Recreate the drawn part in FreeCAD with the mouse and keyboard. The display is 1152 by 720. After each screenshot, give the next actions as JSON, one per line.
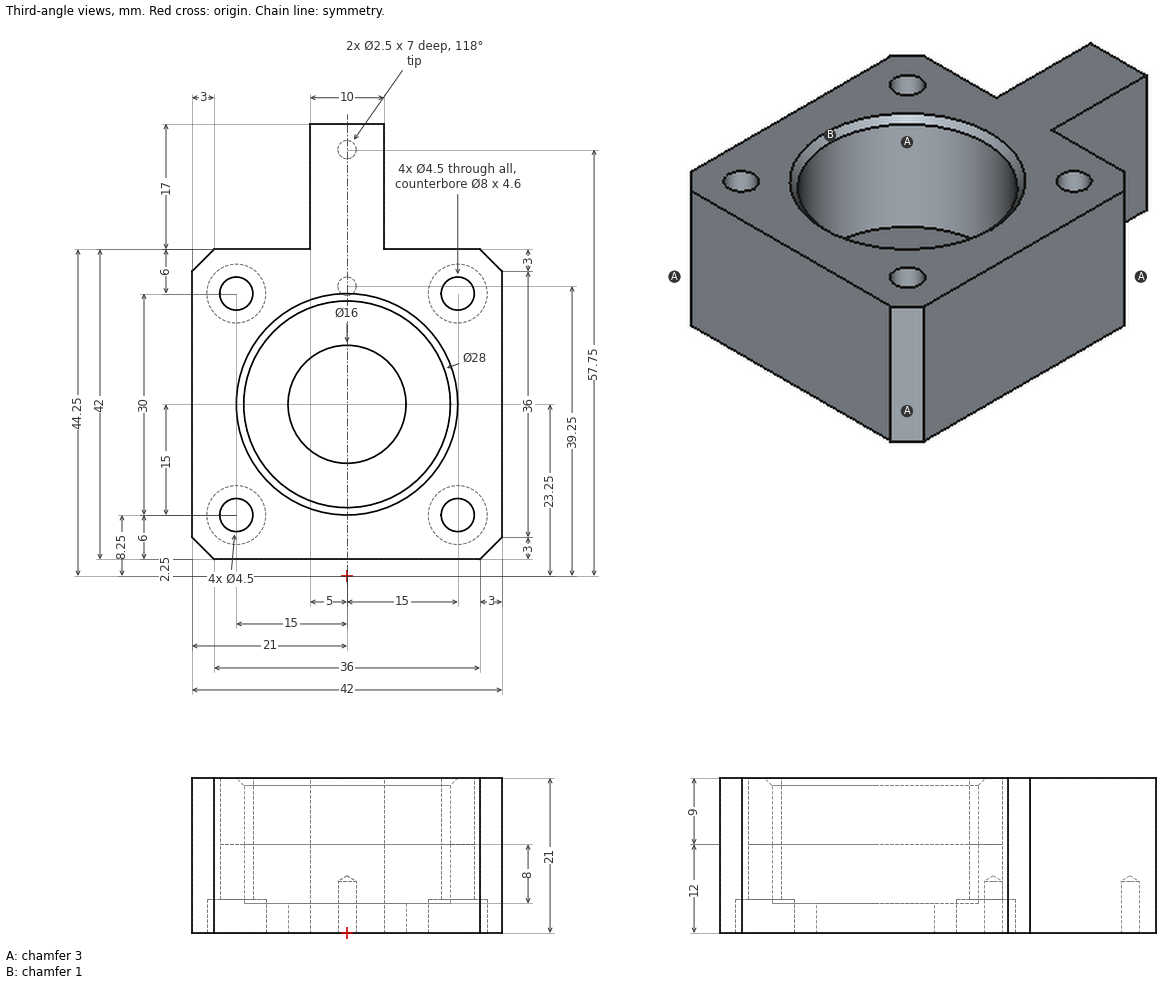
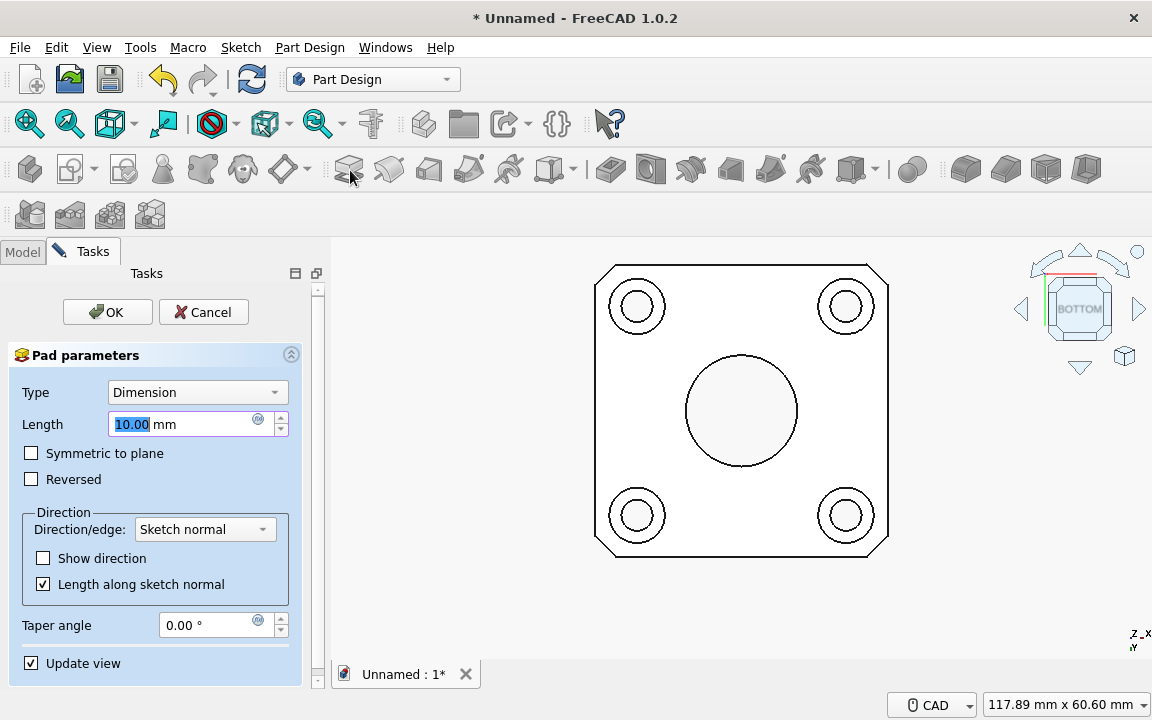
{"action": "type", "text": "21"}
{"action": "key", "text": "Tab"}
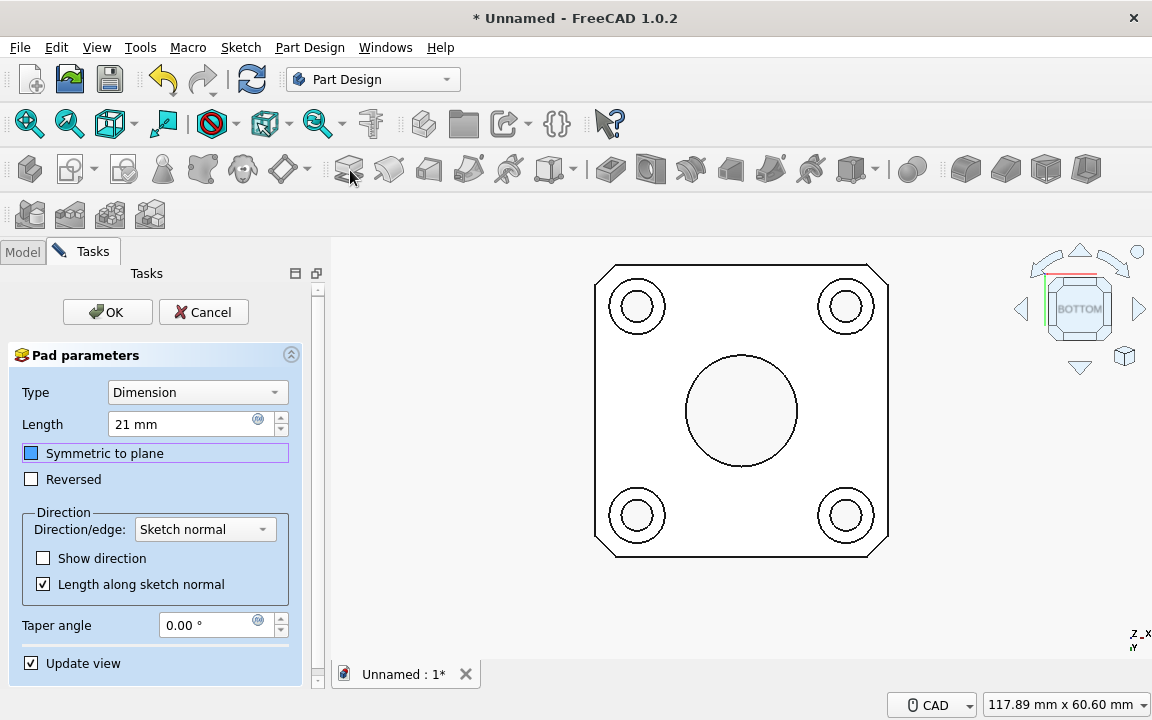
{"action": "left_click", "coordinate": [30, 479]}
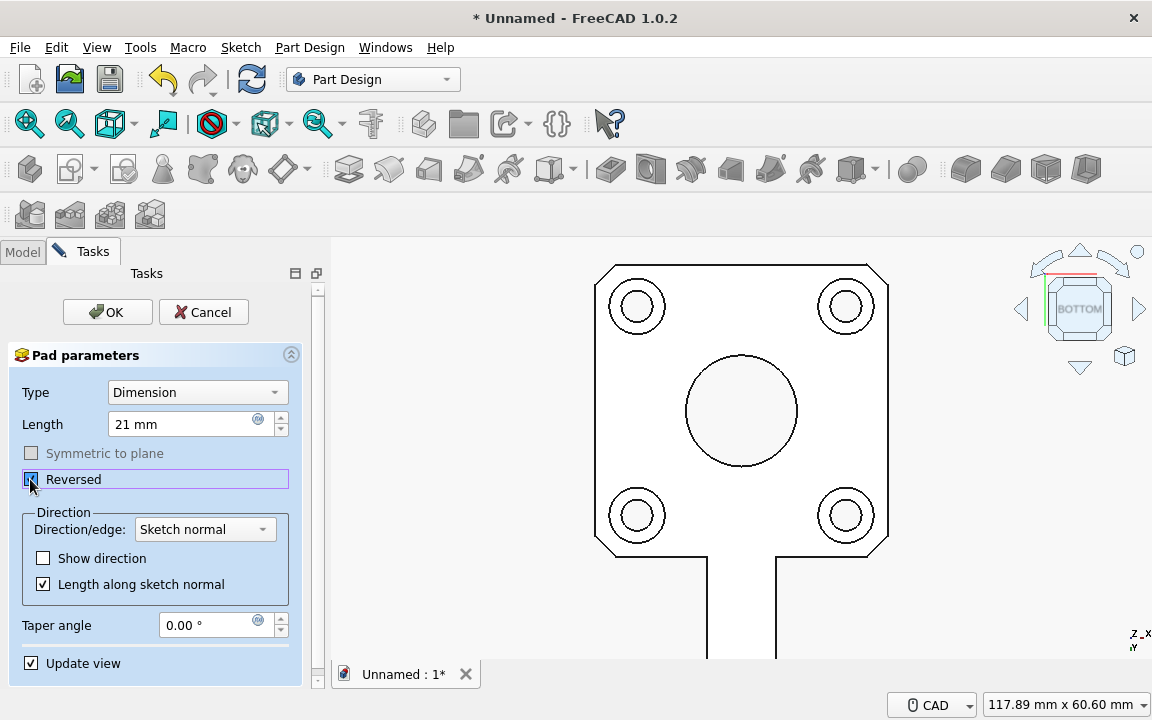
{"action": "left_click", "coordinate": [108, 312]}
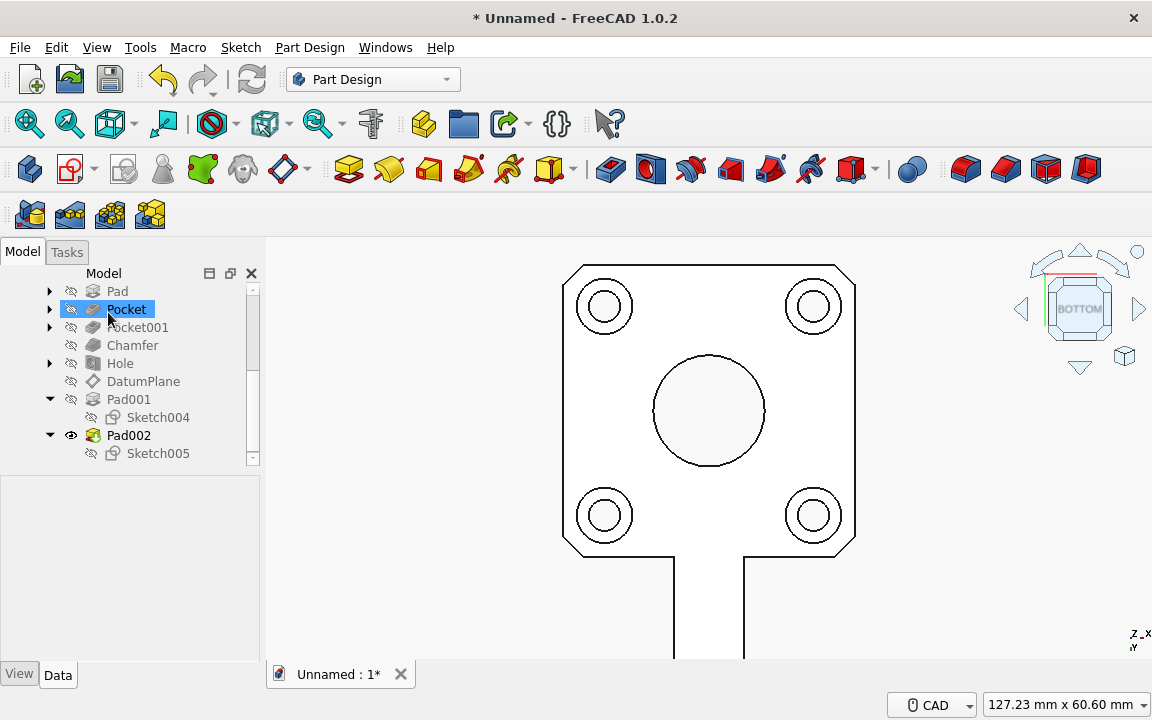
{"action": "left_click", "coordinate": [30, 124]}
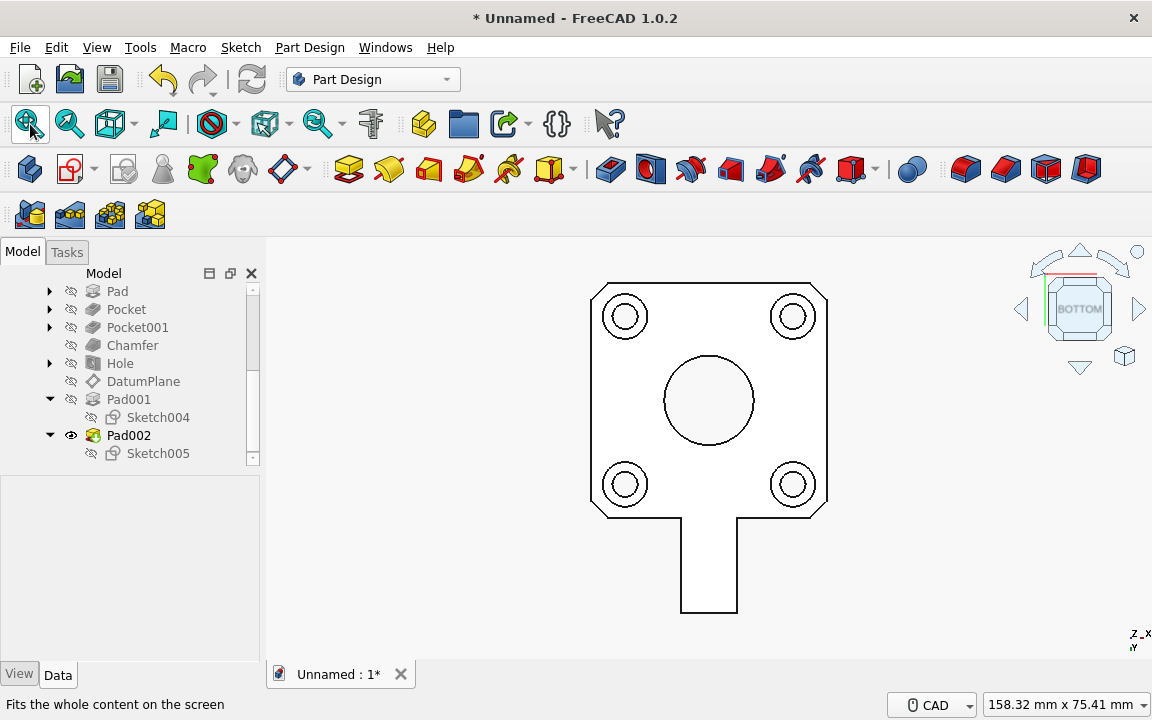
{"action": "left_click", "coordinate": [709, 494]}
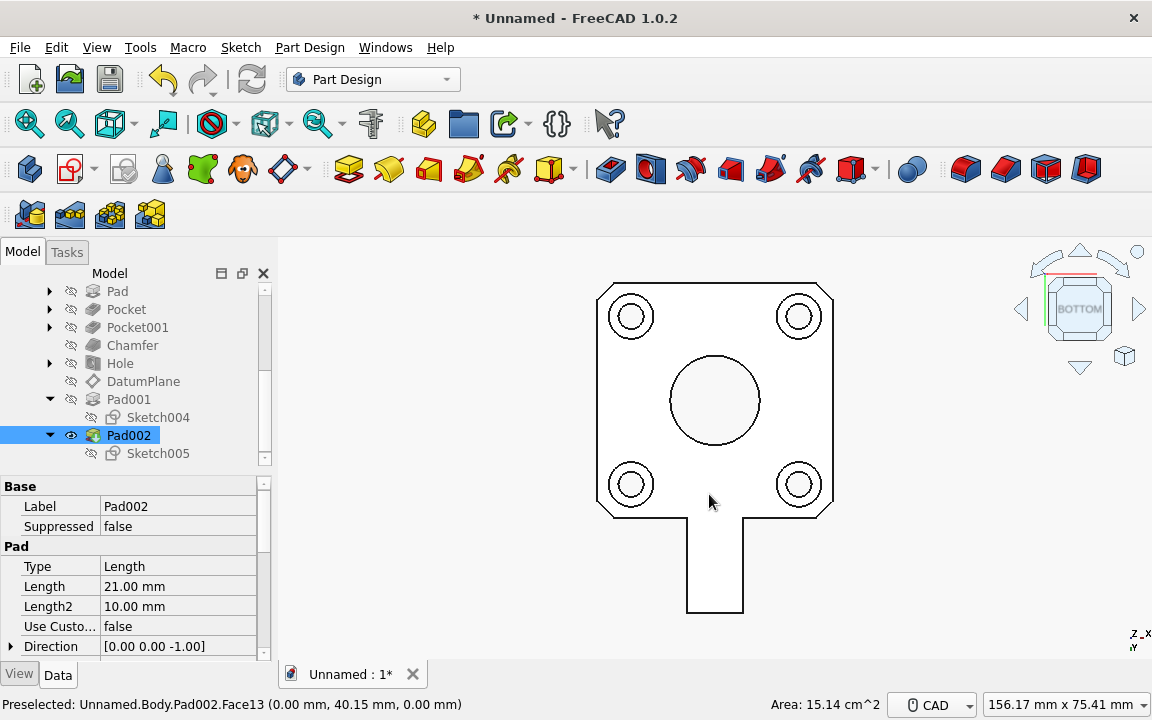
{"action": "left_click", "coordinate": [70, 170]}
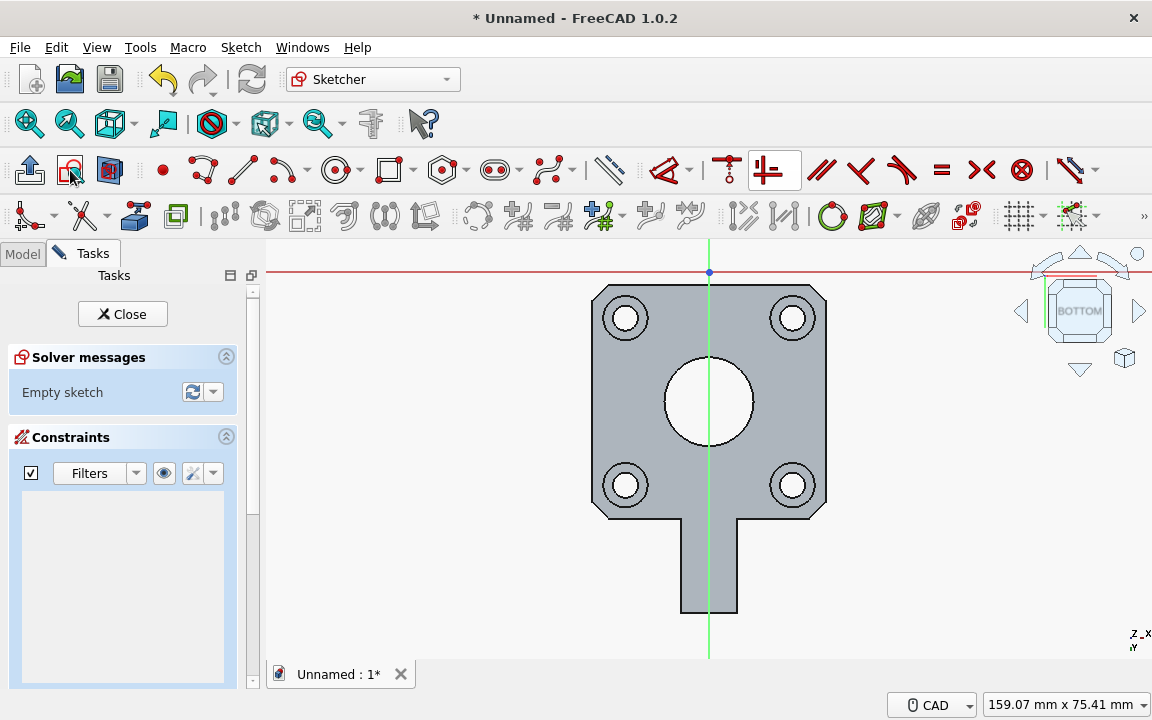
{"action": "scroll", "coordinate": [765, 618], "scroll_direction": "up", "scroll_amount": 4}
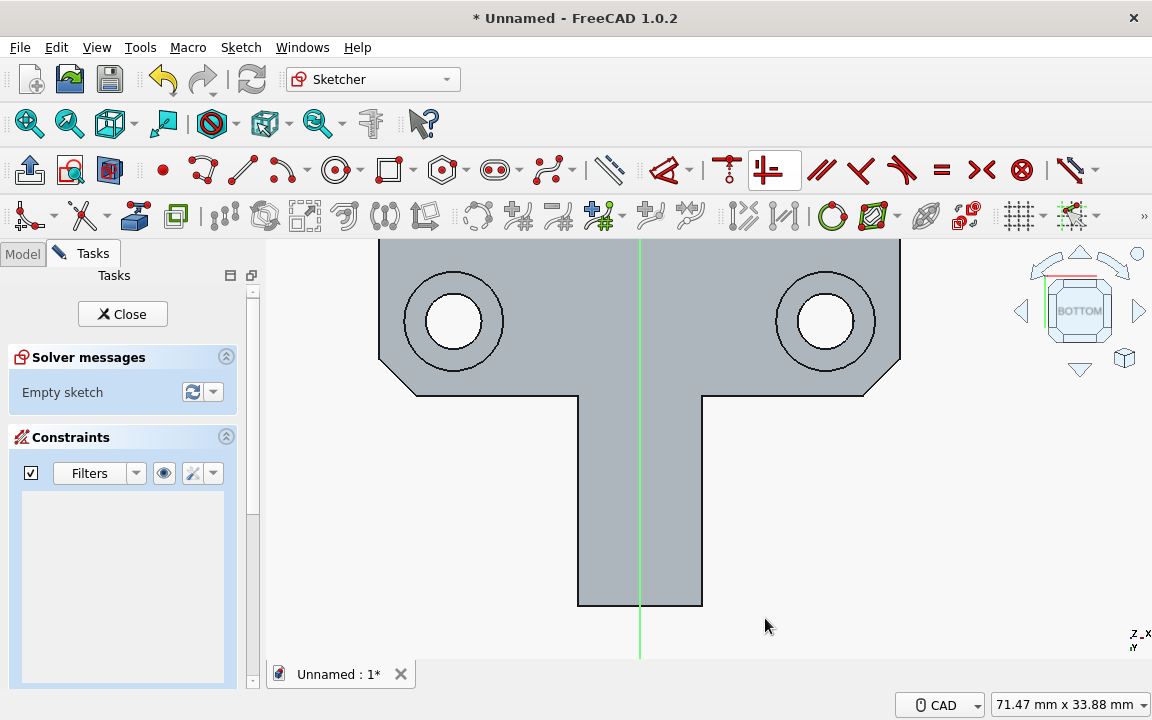
{"action": "left_click", "coordinate": [336, 170]}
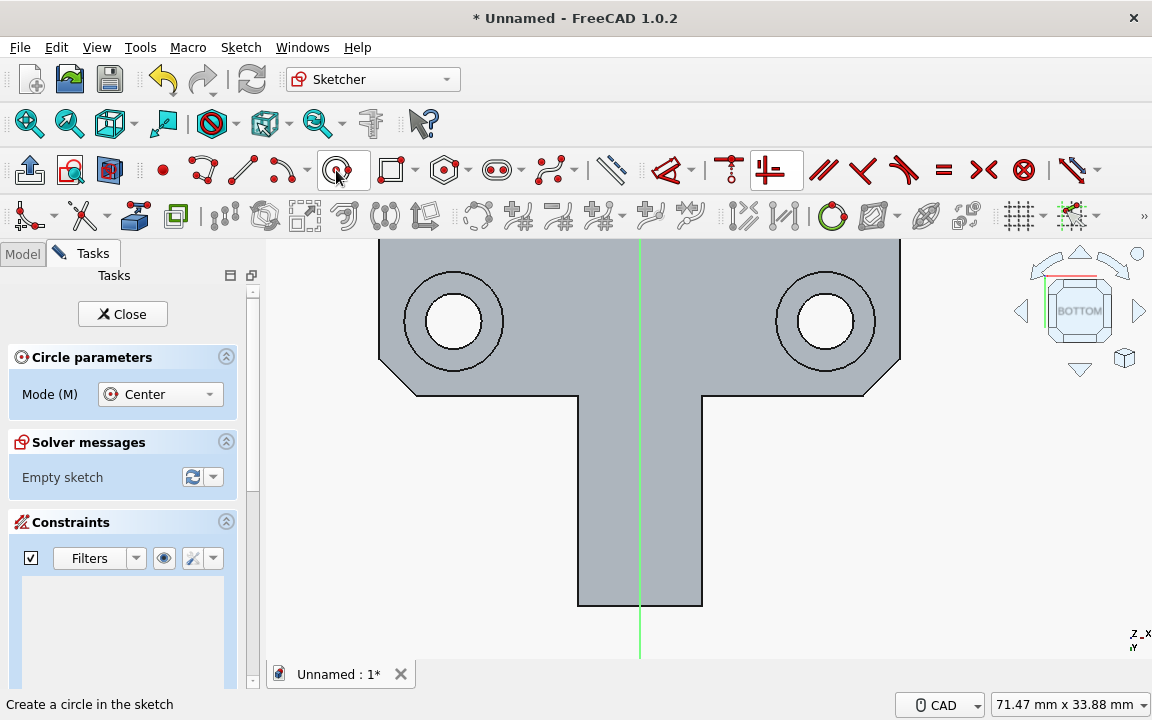
{"action": "scroll", "coordinate": [640, 563], "scroll_direction": "up", "scroll_amount": 2}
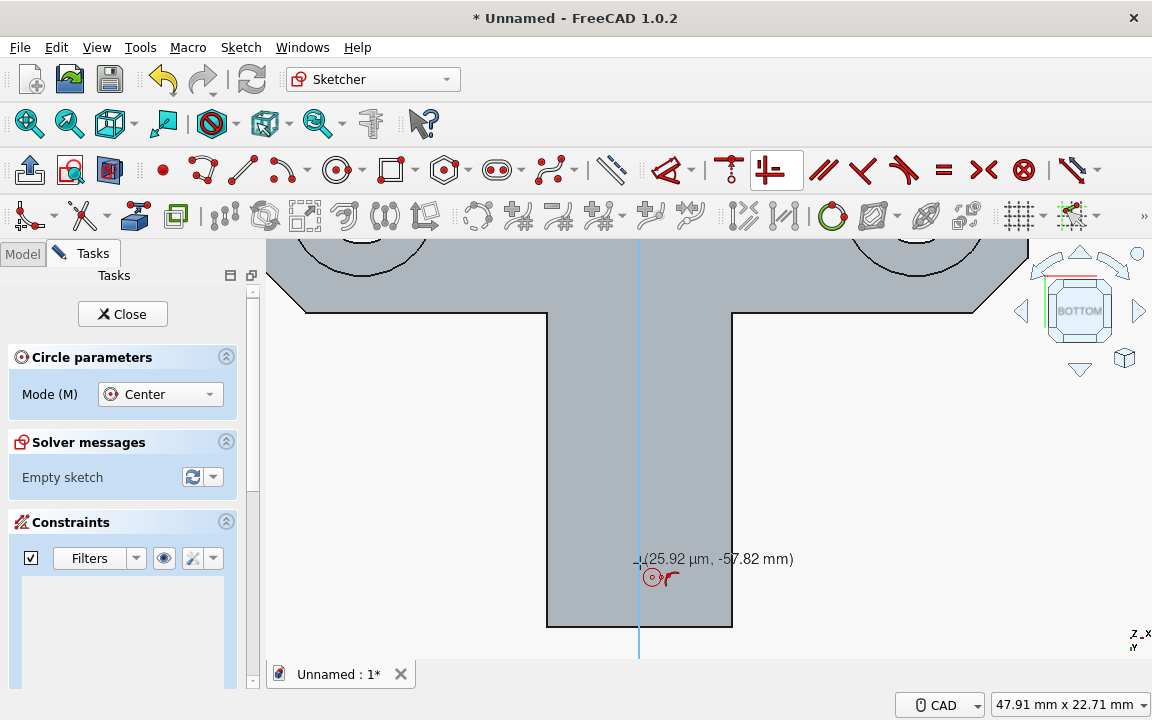
{"action": "left_click", "coordinate": [639, 563]}
{"action": "left_click", "coordinate": [656, 546]}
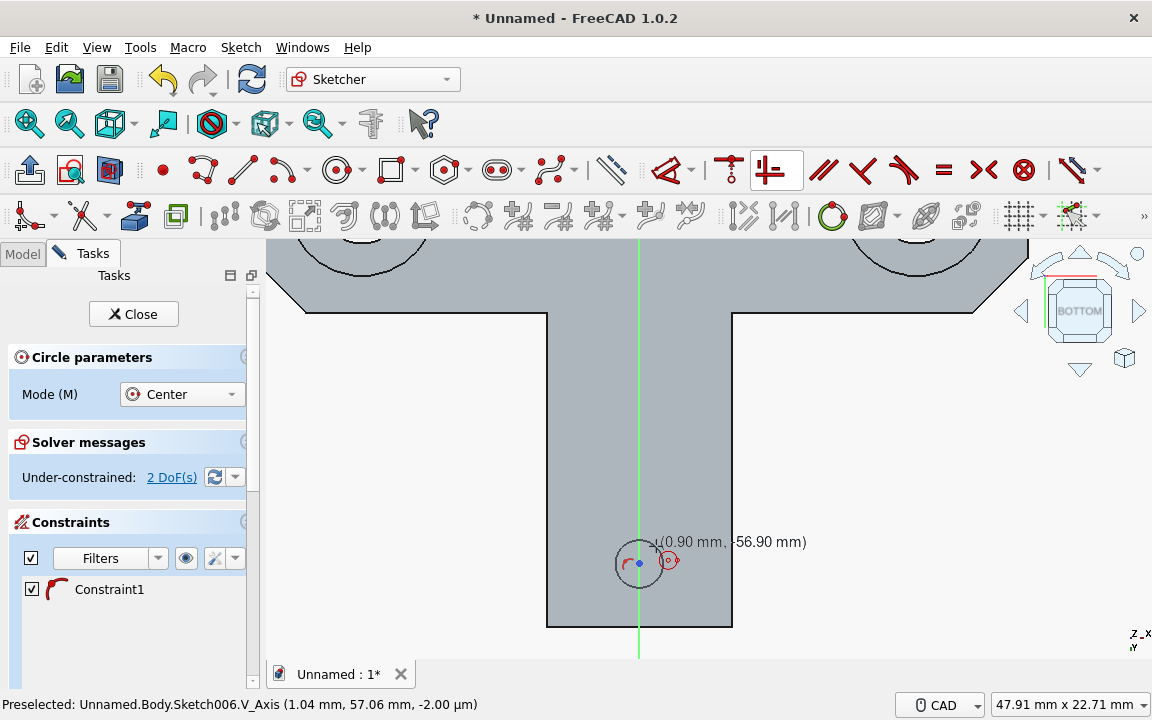
{"action": "scroll", "coordinate": [643, 566], "scroll_direction": "down", "scroll_amount": 2}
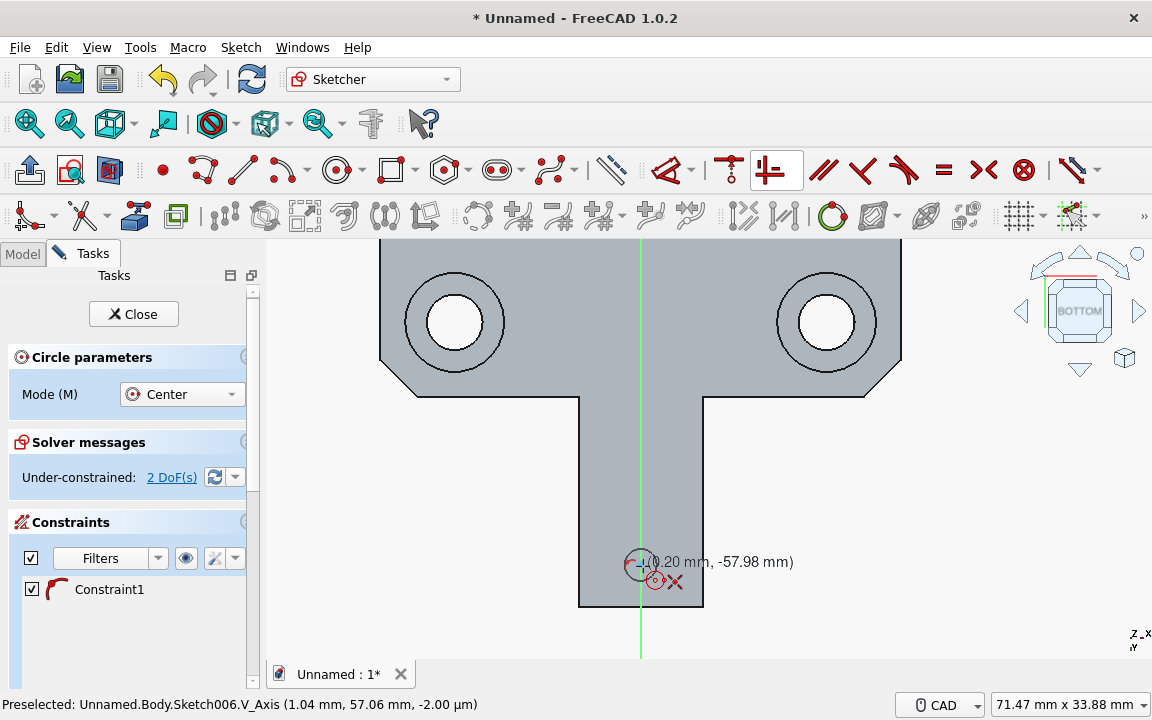
{"action": "scroll", "coordinate": [641, 335], "scroll_direction": "up", "scroll_amount": 2}